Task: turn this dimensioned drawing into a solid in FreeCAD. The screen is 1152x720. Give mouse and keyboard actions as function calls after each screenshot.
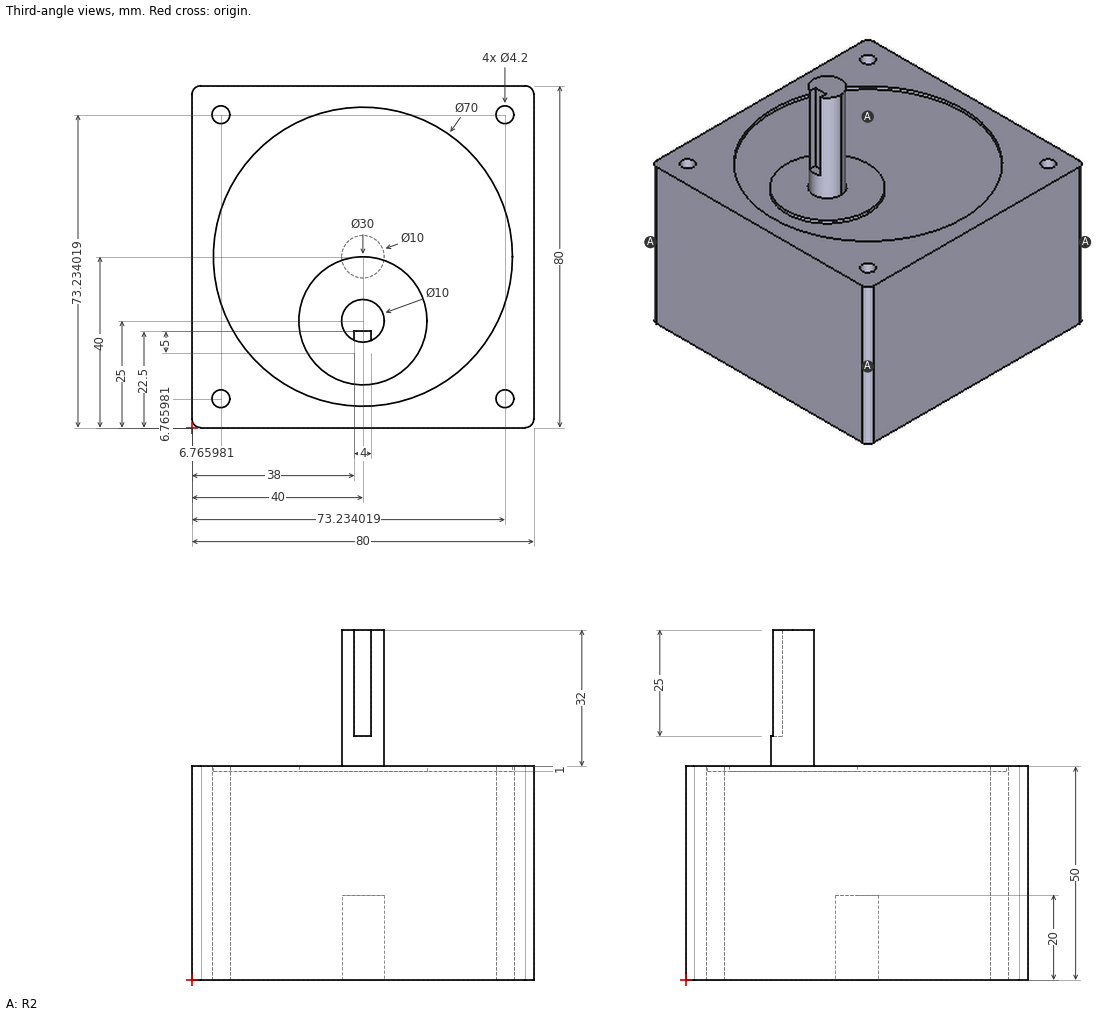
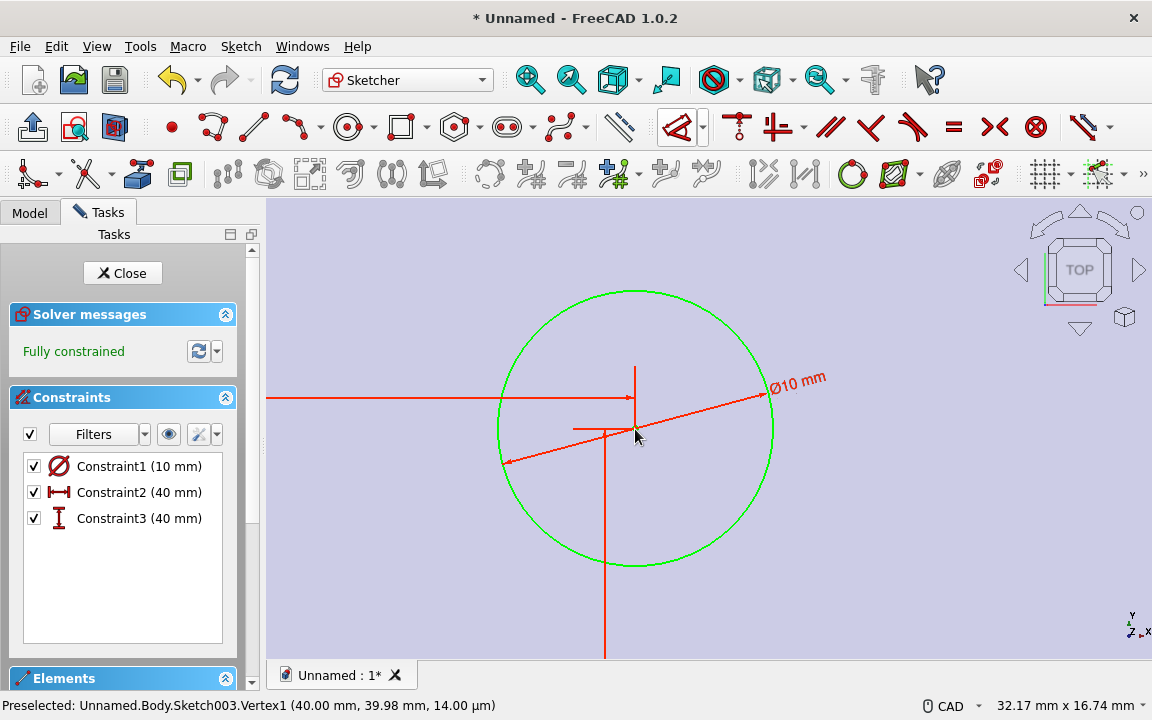
click(123, 273)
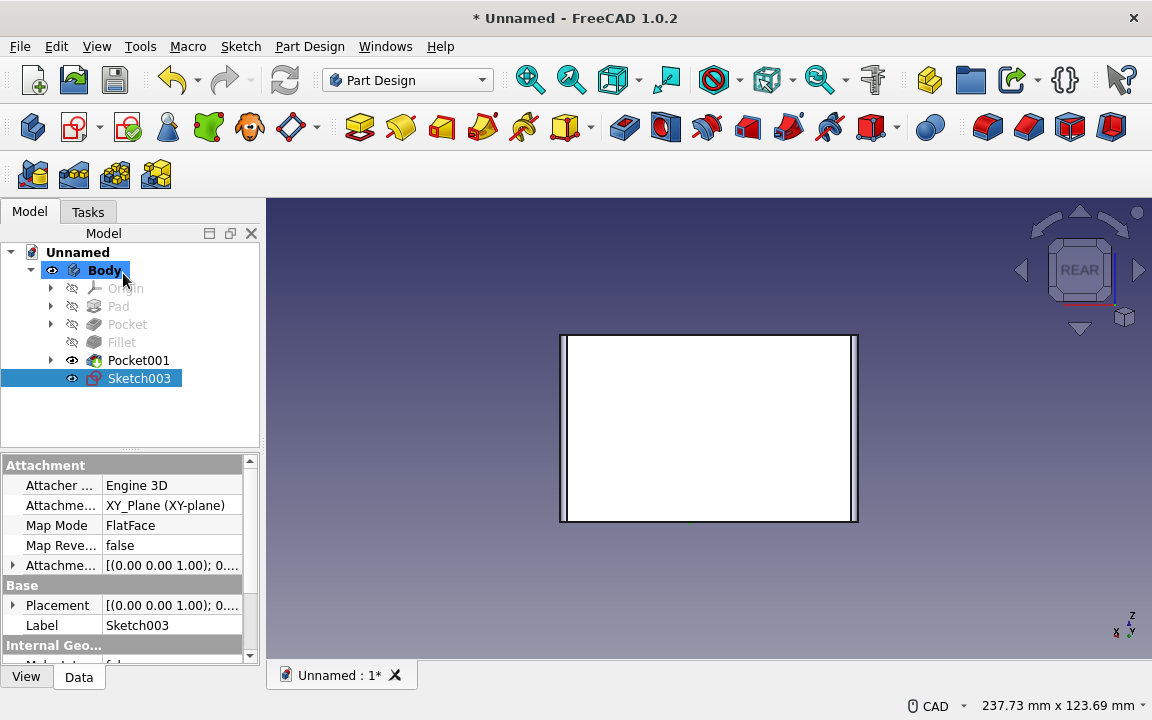
click(625, 128)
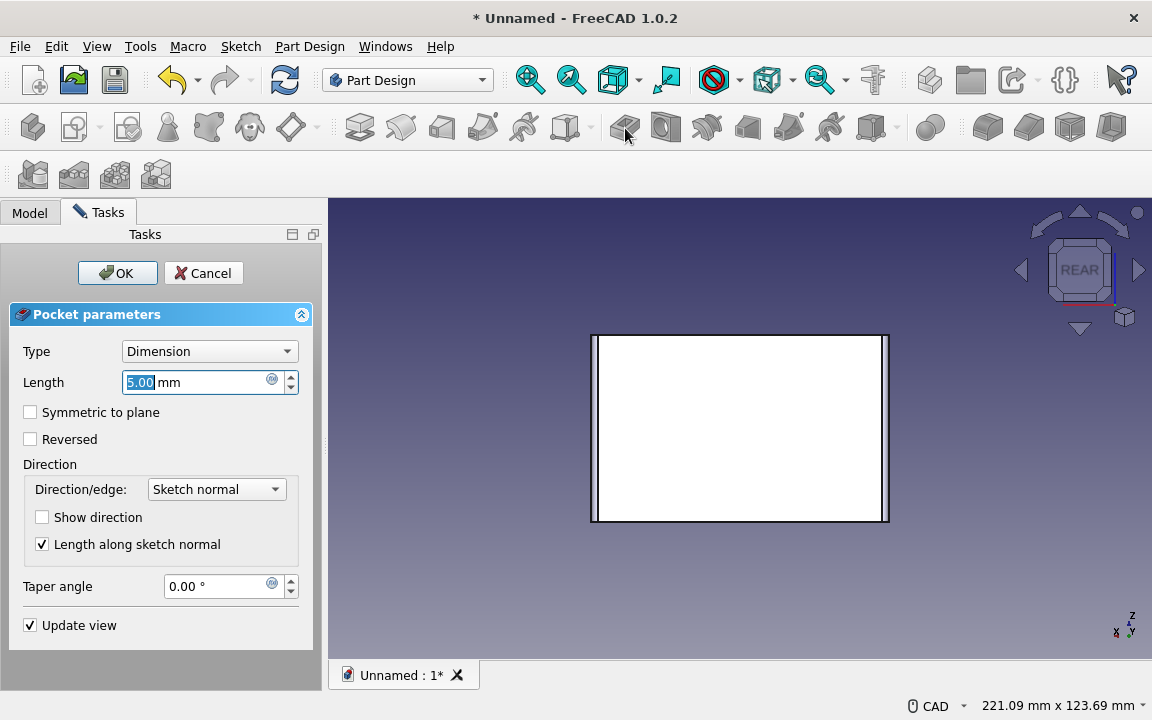
text(20)
key(Tab)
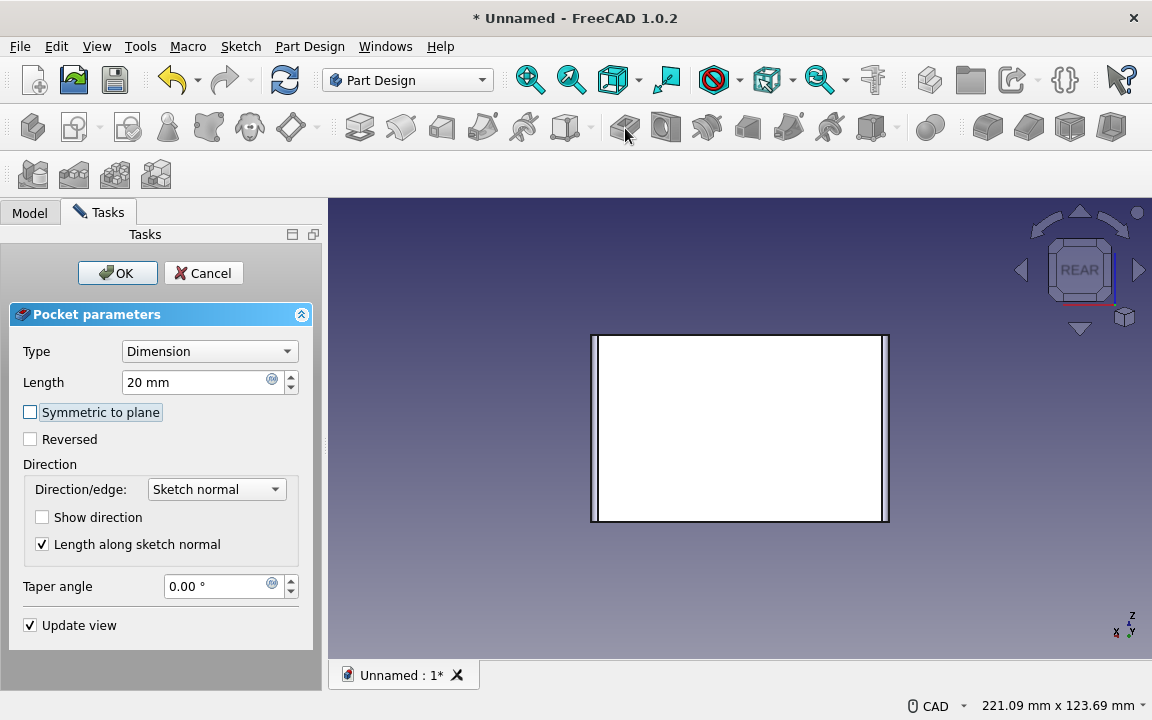
click(31, 439)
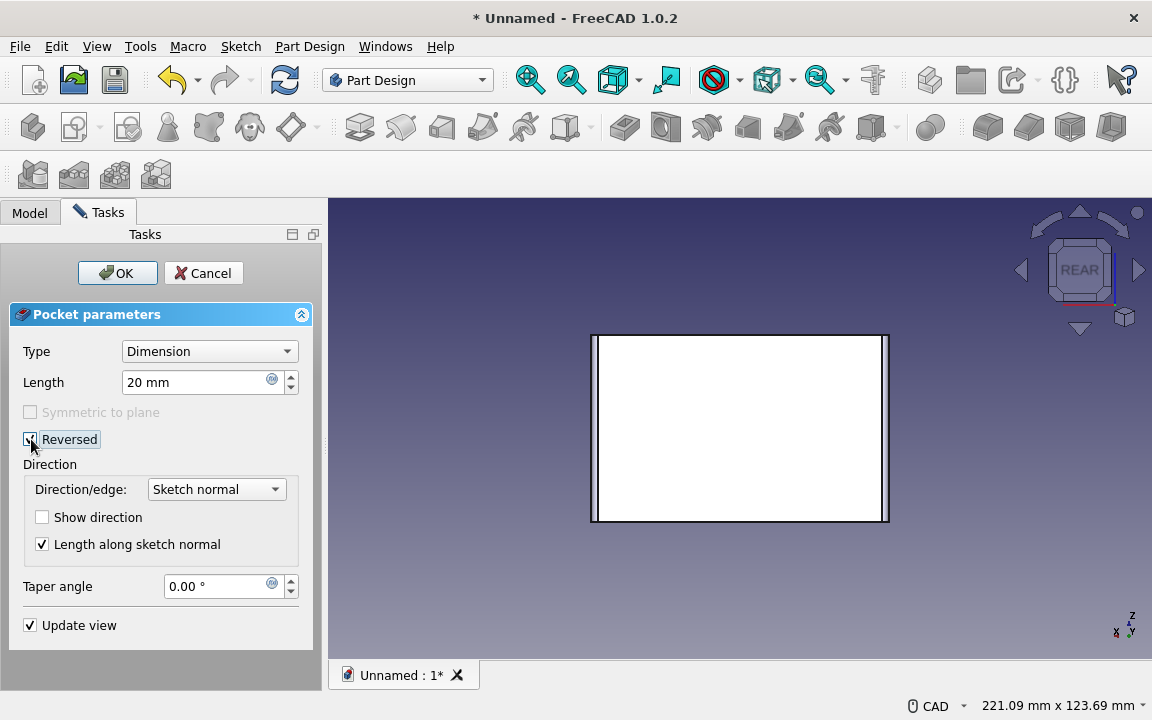
click(118, 273)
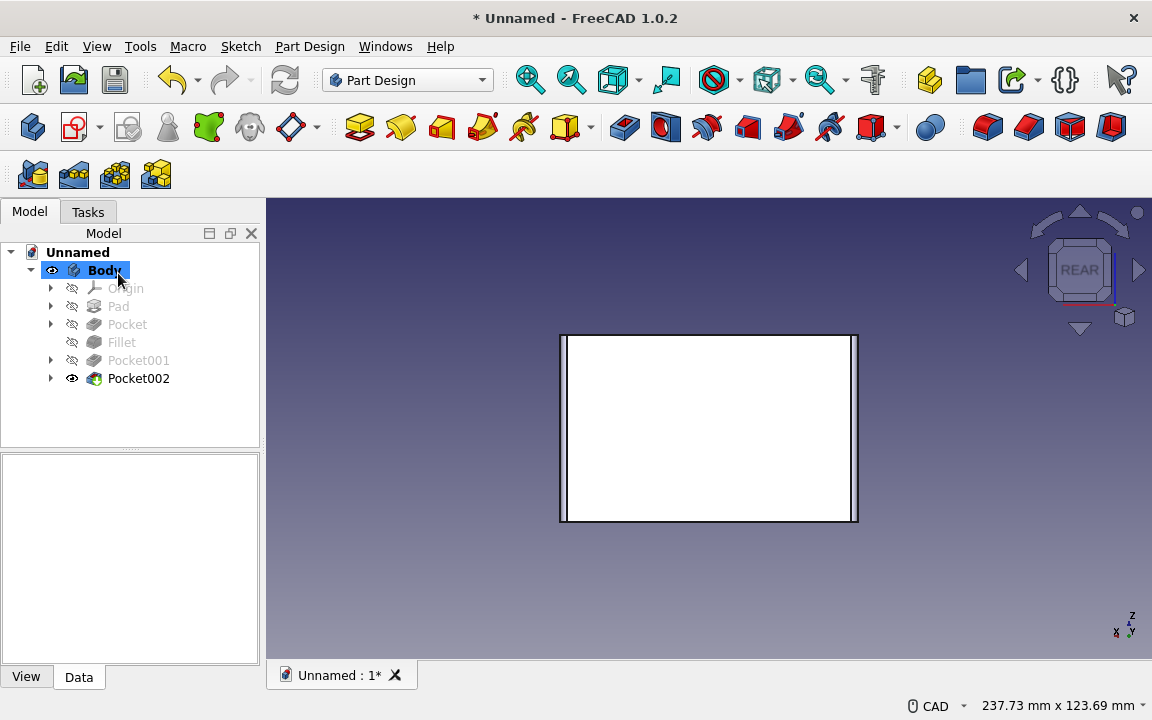
key(v)
key(f)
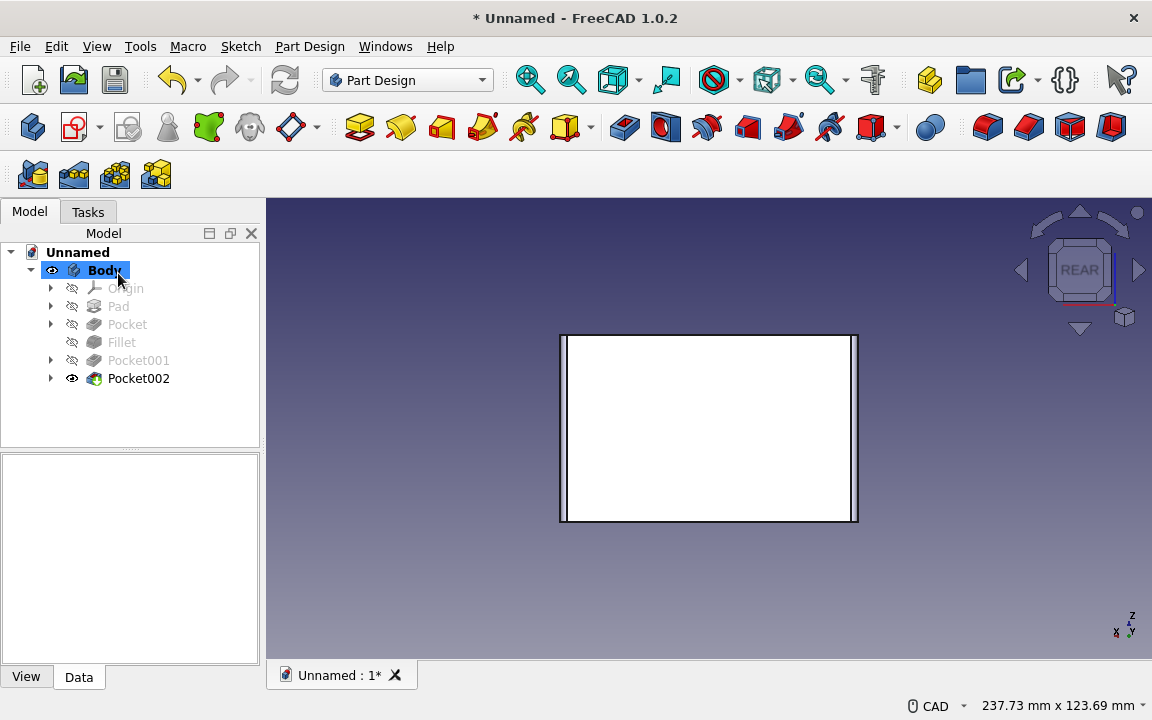
click(33, 128)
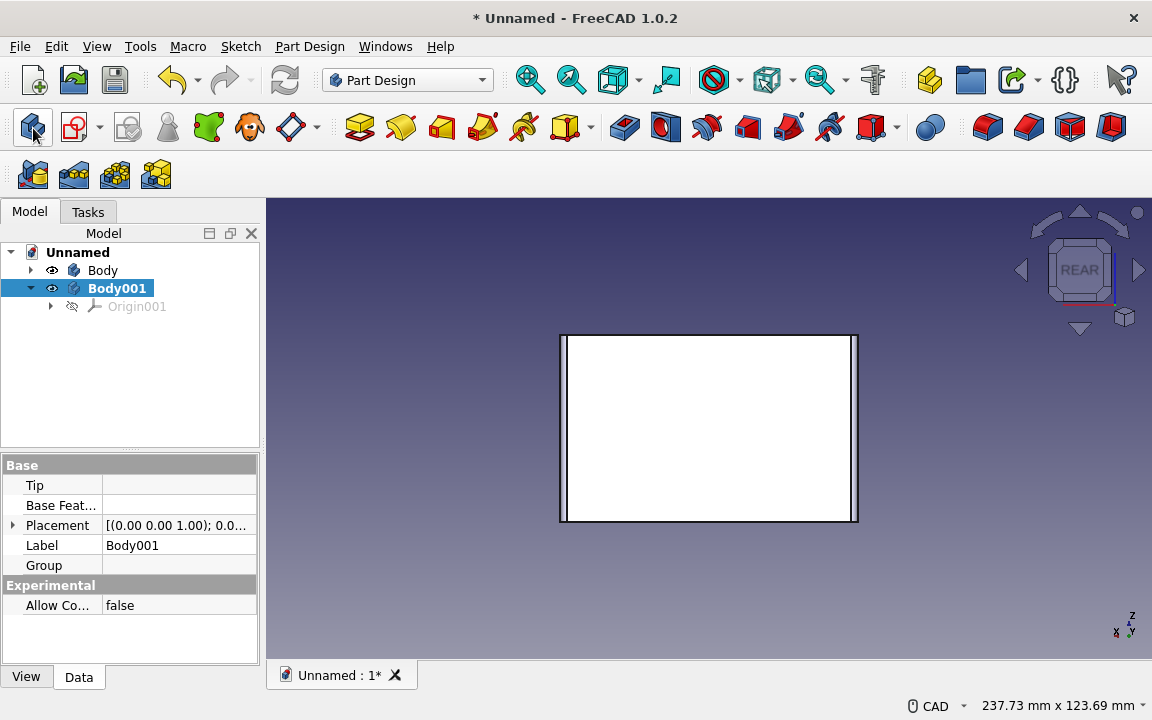
click(51, 306)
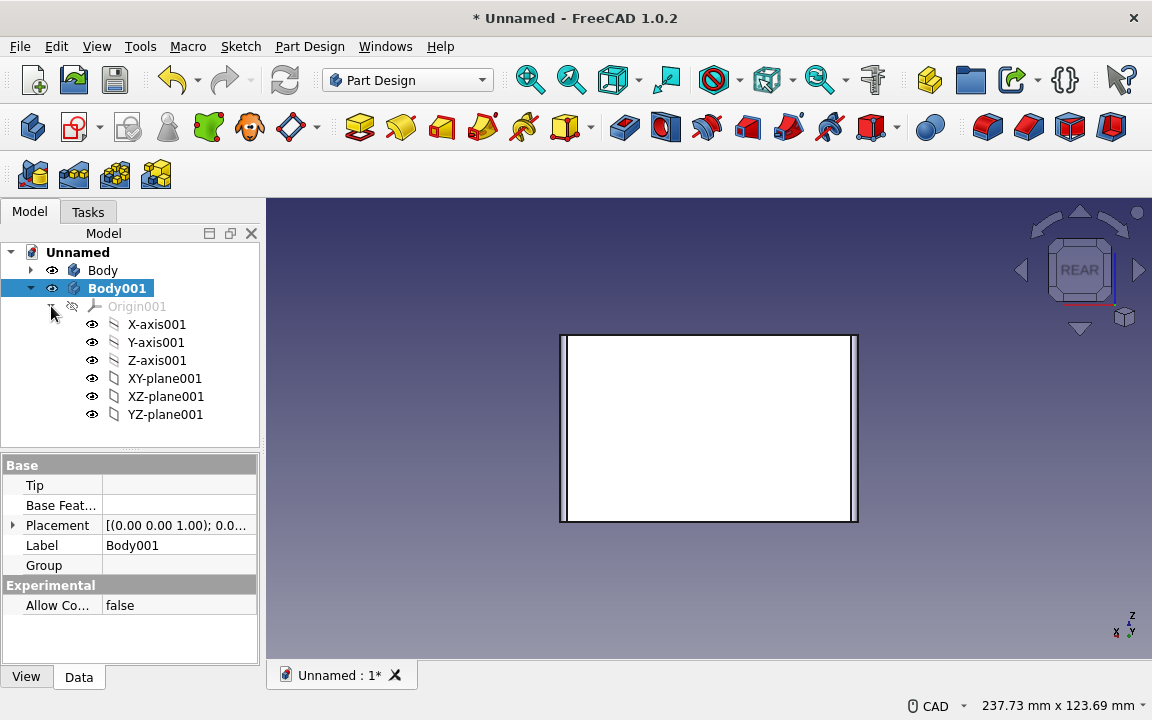
click(137, 378)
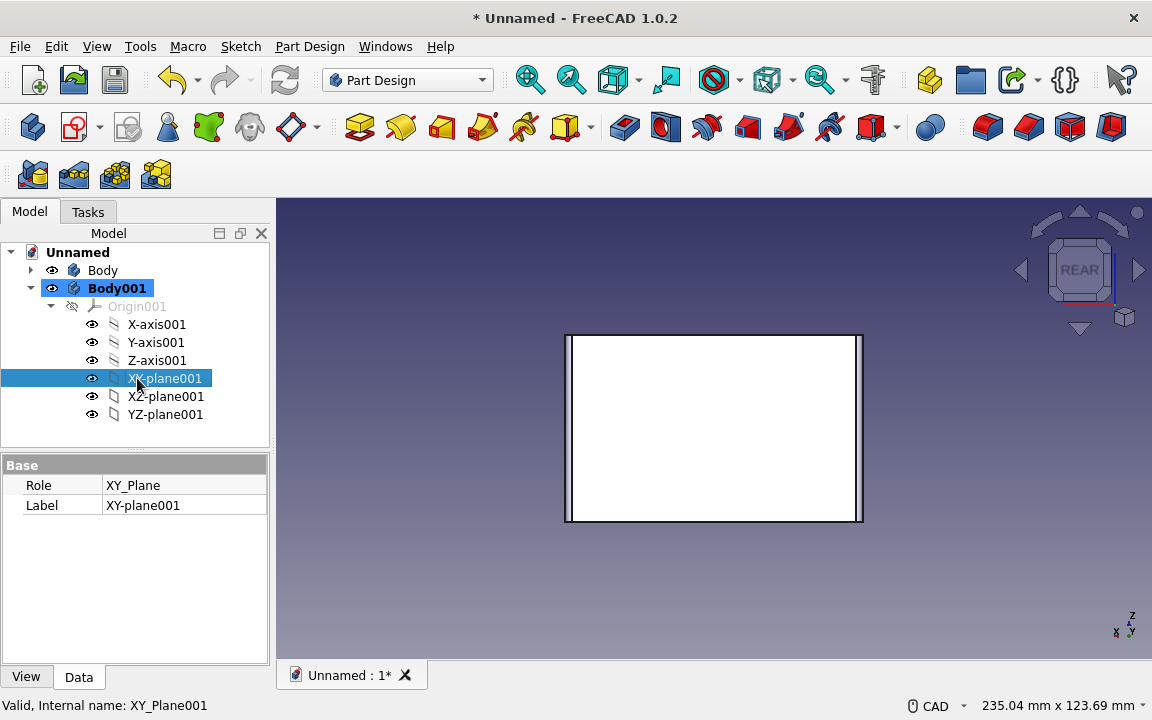
click(290, 128)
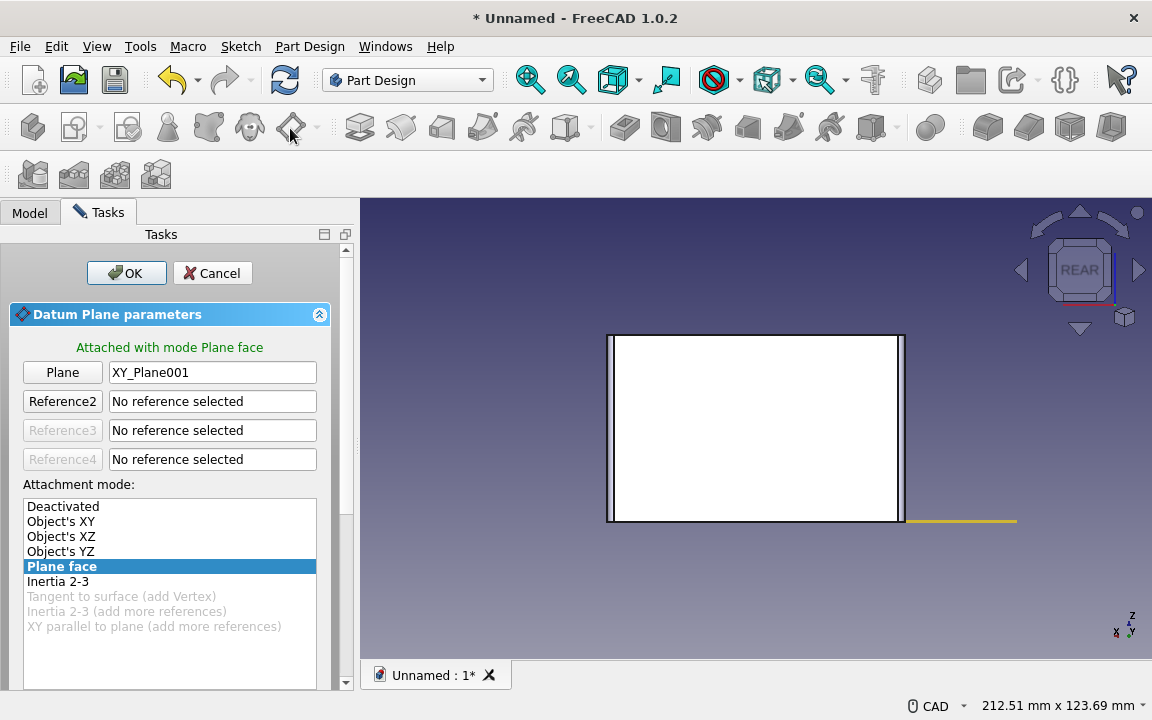
scroll(346, 467, down, 4)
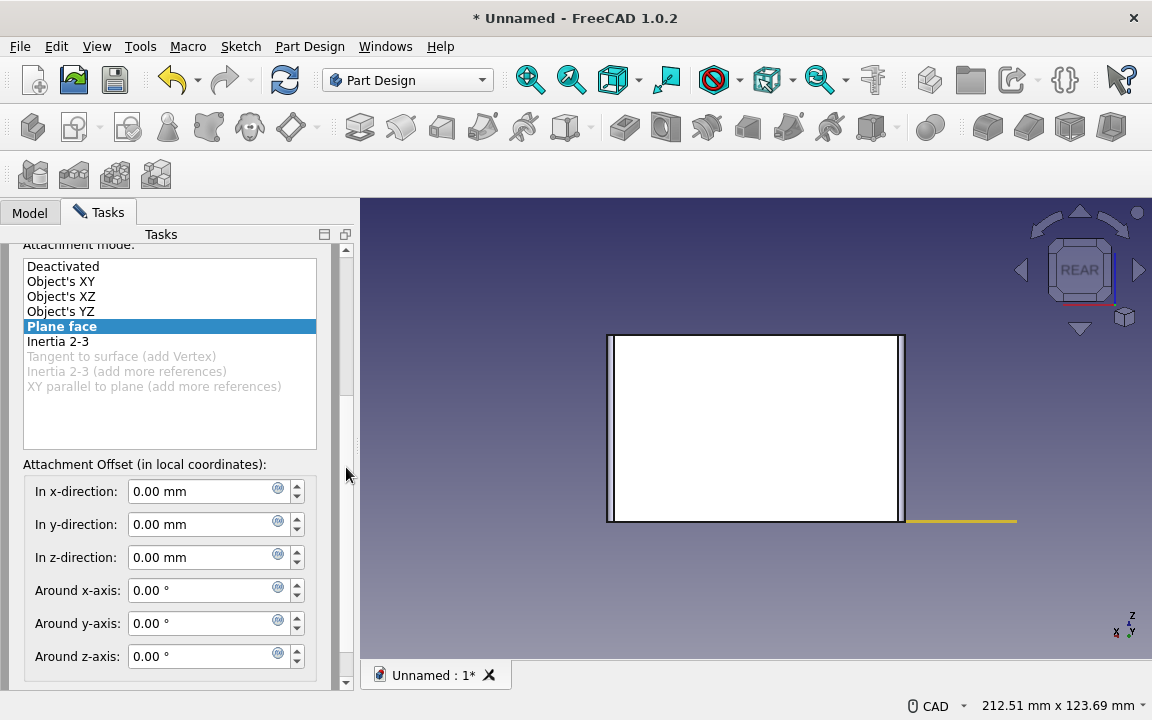
triple_click(210, 558)